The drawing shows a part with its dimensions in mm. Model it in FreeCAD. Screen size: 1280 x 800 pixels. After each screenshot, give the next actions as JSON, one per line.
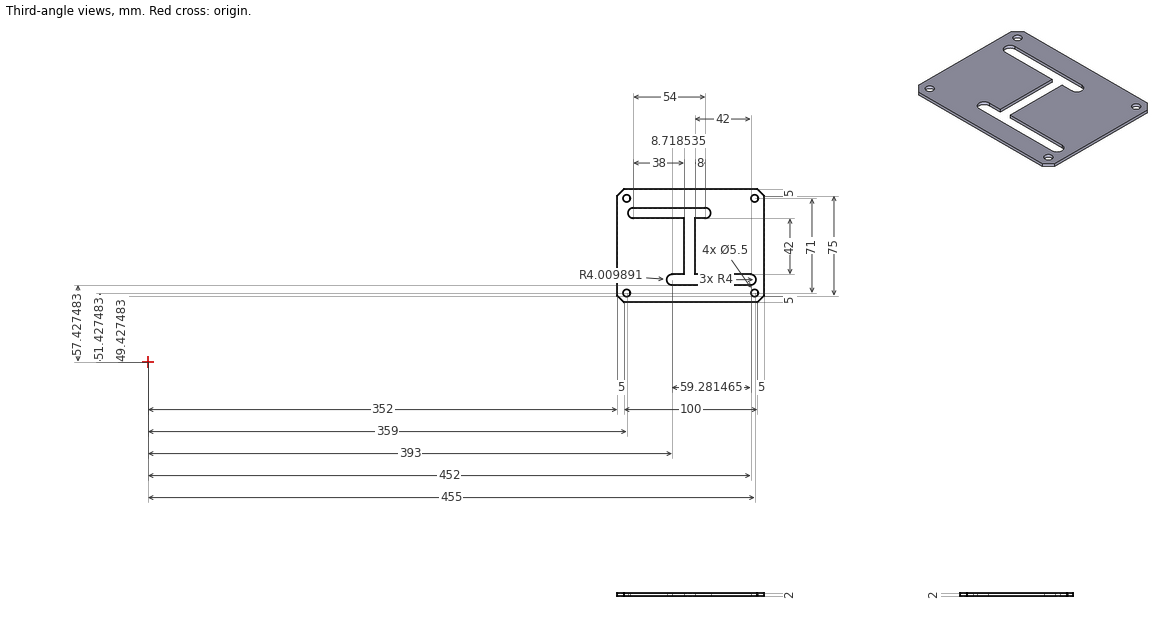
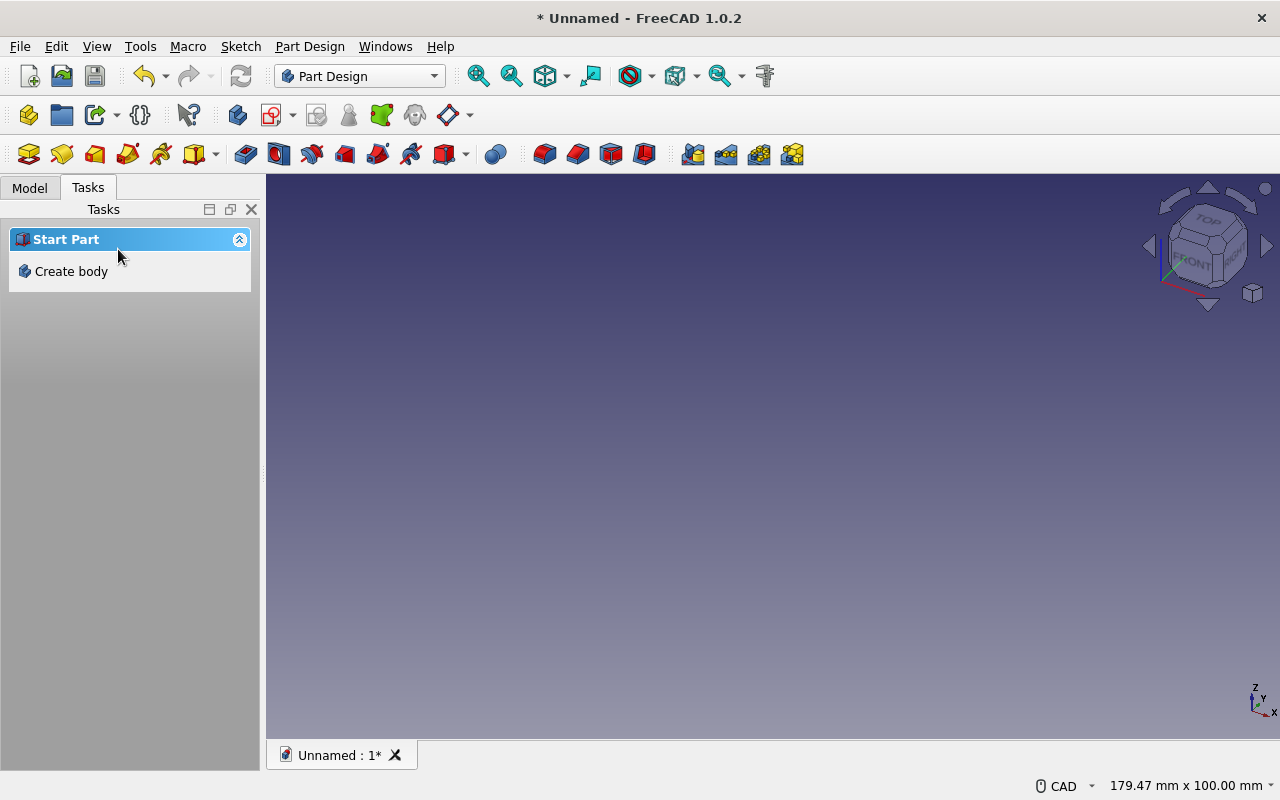
{"action": "key", "text": "v f"}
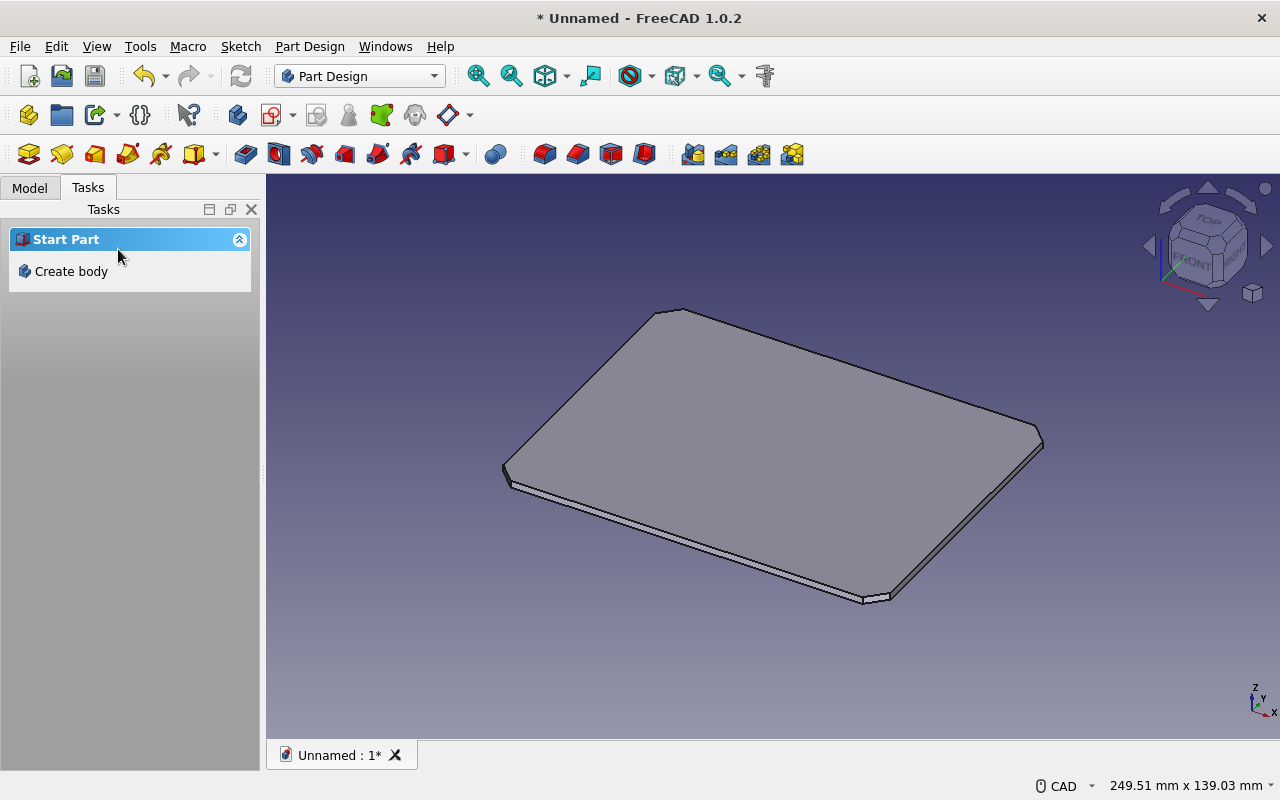
{"action": "left_click", "coordinate": [773, 452]}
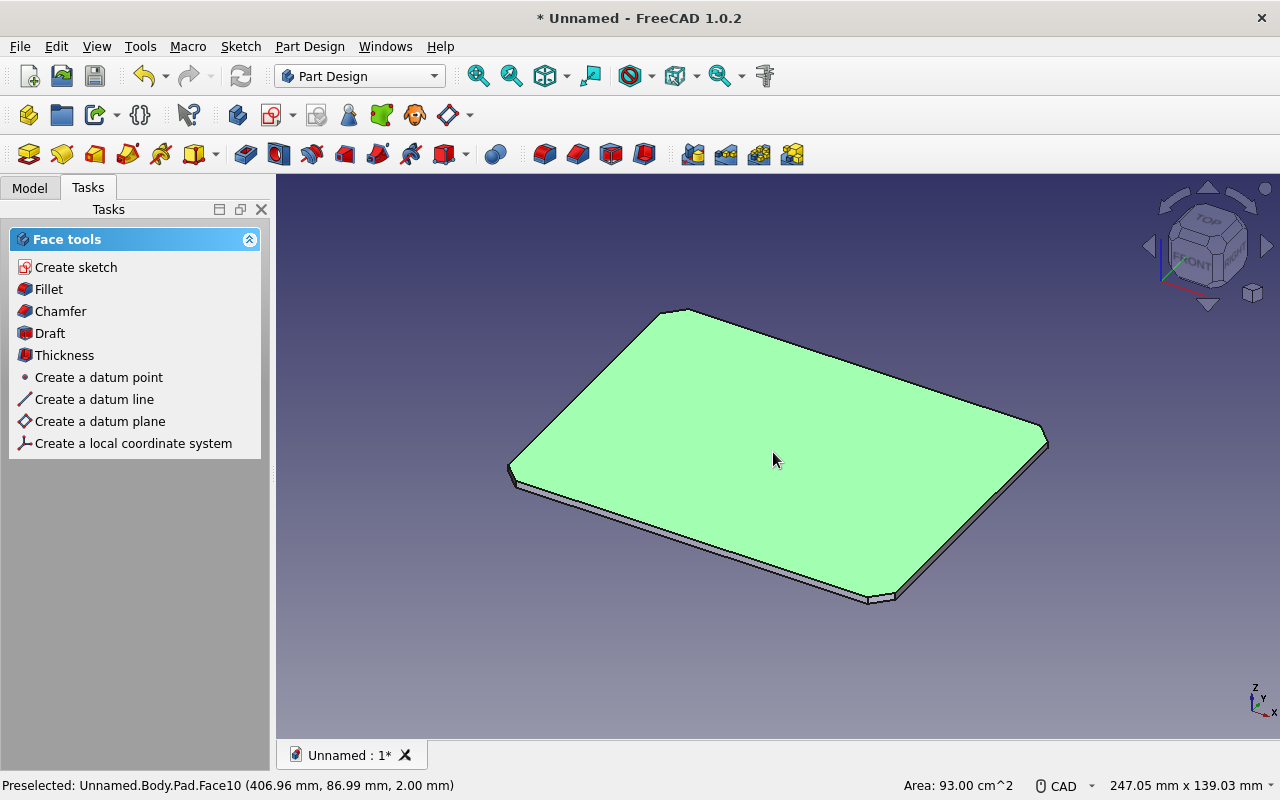
{"action": "left_click", "coordinate": [270, 116]}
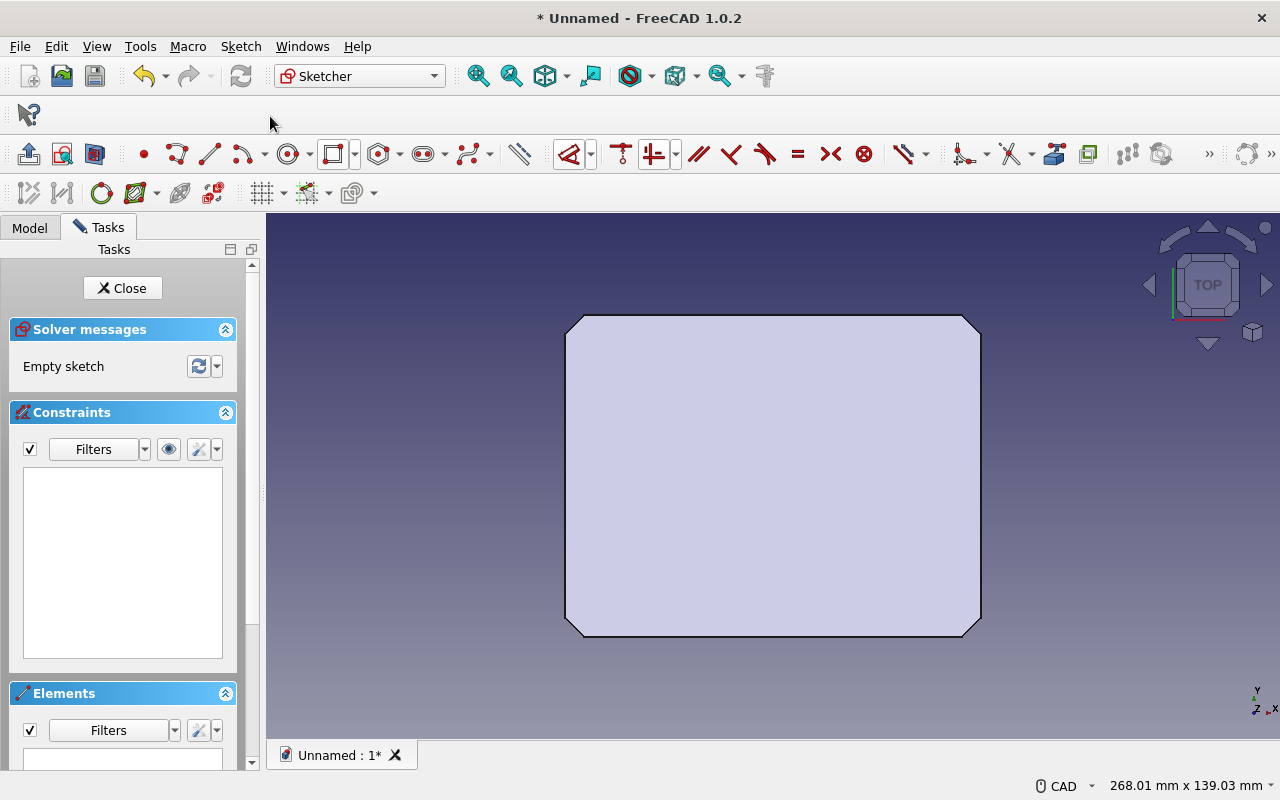
{"action": "scroll", "coordinate": [924, 482], "scroll_direction": "up", "scroll_amount": 2}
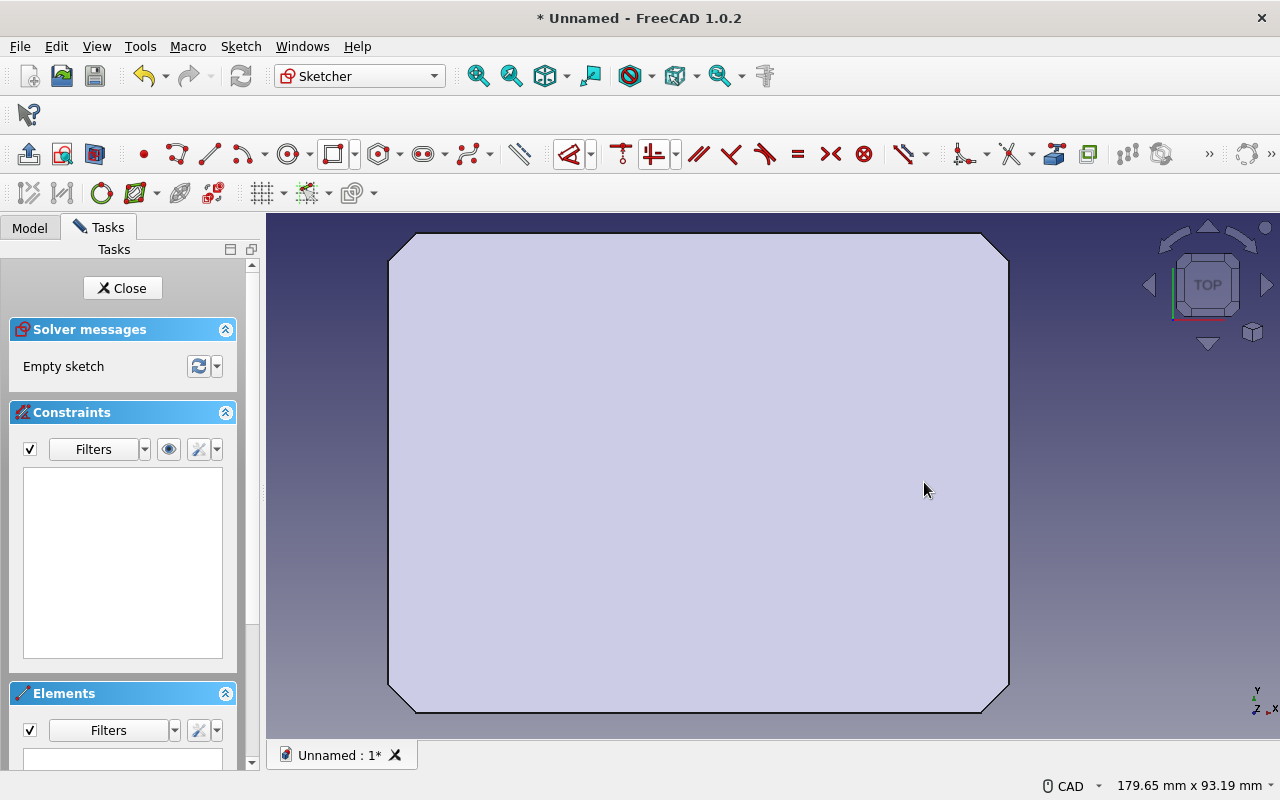
{"action": "left_click", "coordinate": [210, 154]}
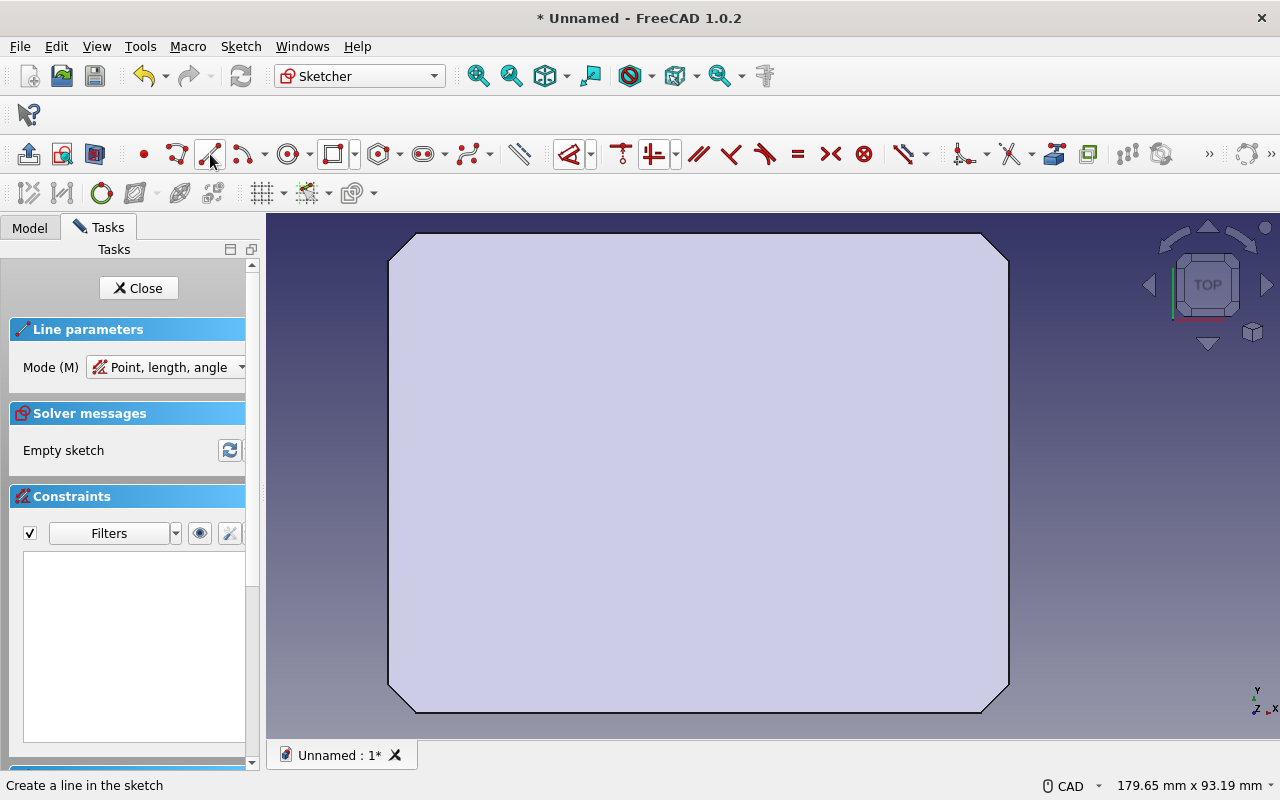
{"action": "left_click", "coordinate": [618, 639]}
{"action": "left_click", "coordinate": [952, 639]}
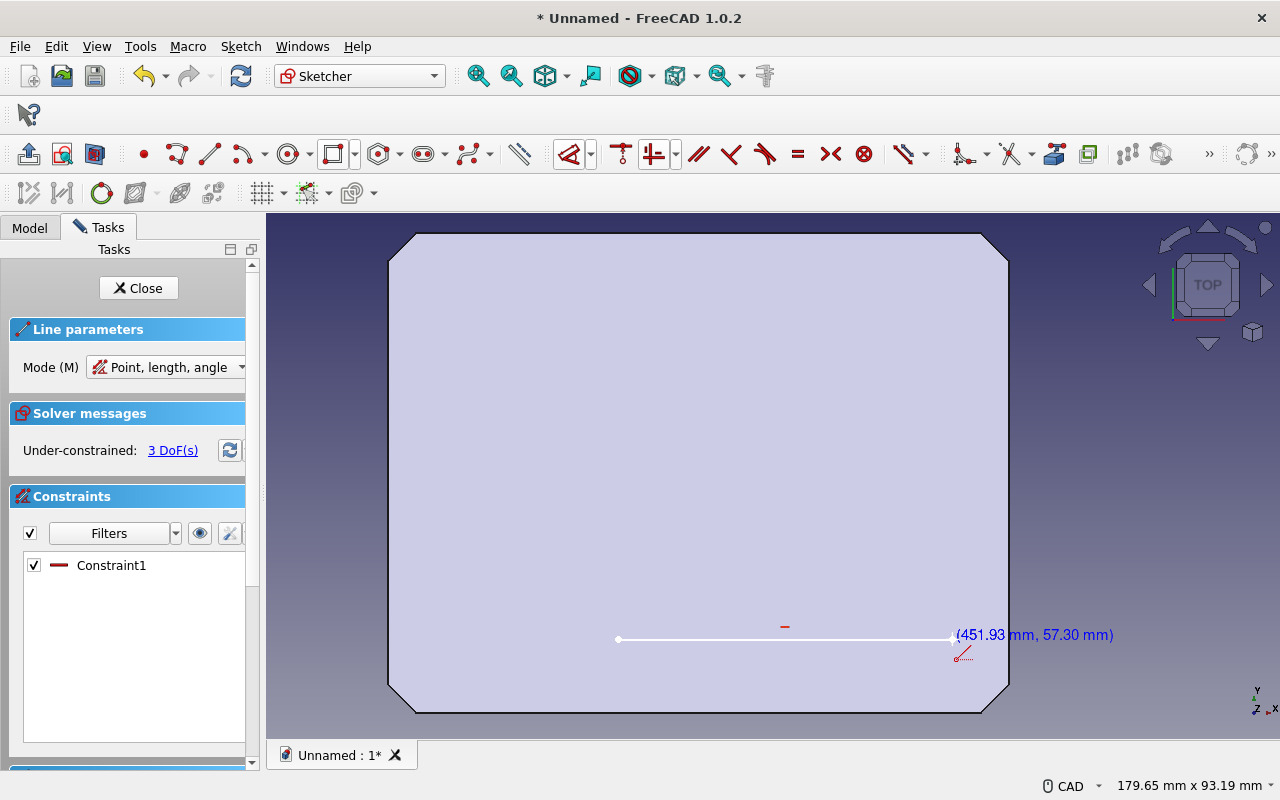
{"action": "left_click", "coordinate": [177, 154]}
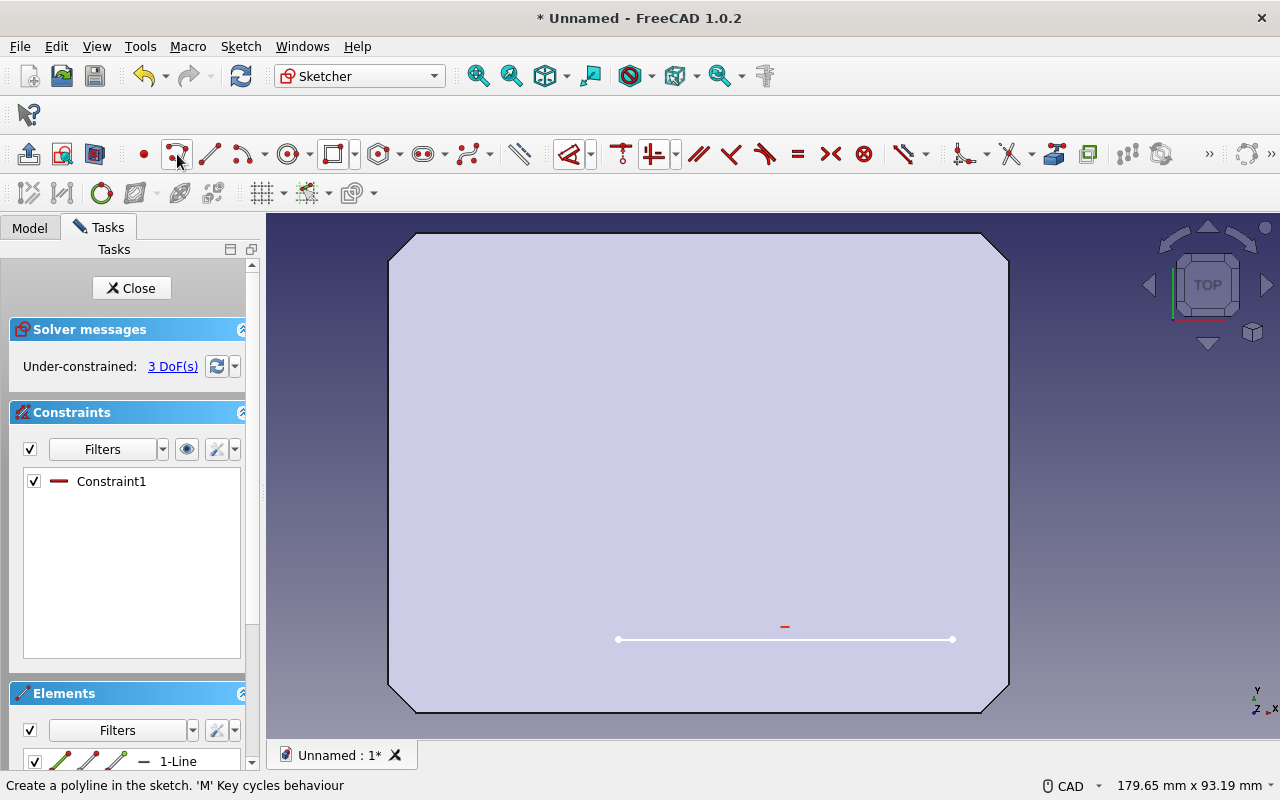
{"action": "left_click", "coordinate": [952, 594]}
{"action": "left_click", "coordinate": [715, 594]}
{"action": "left_click", "coordinate": [715, 357]}
{"action": "left_click", "coordinate": [761, 357]}
{"action": "right_click", "coordinate": [761, 357]}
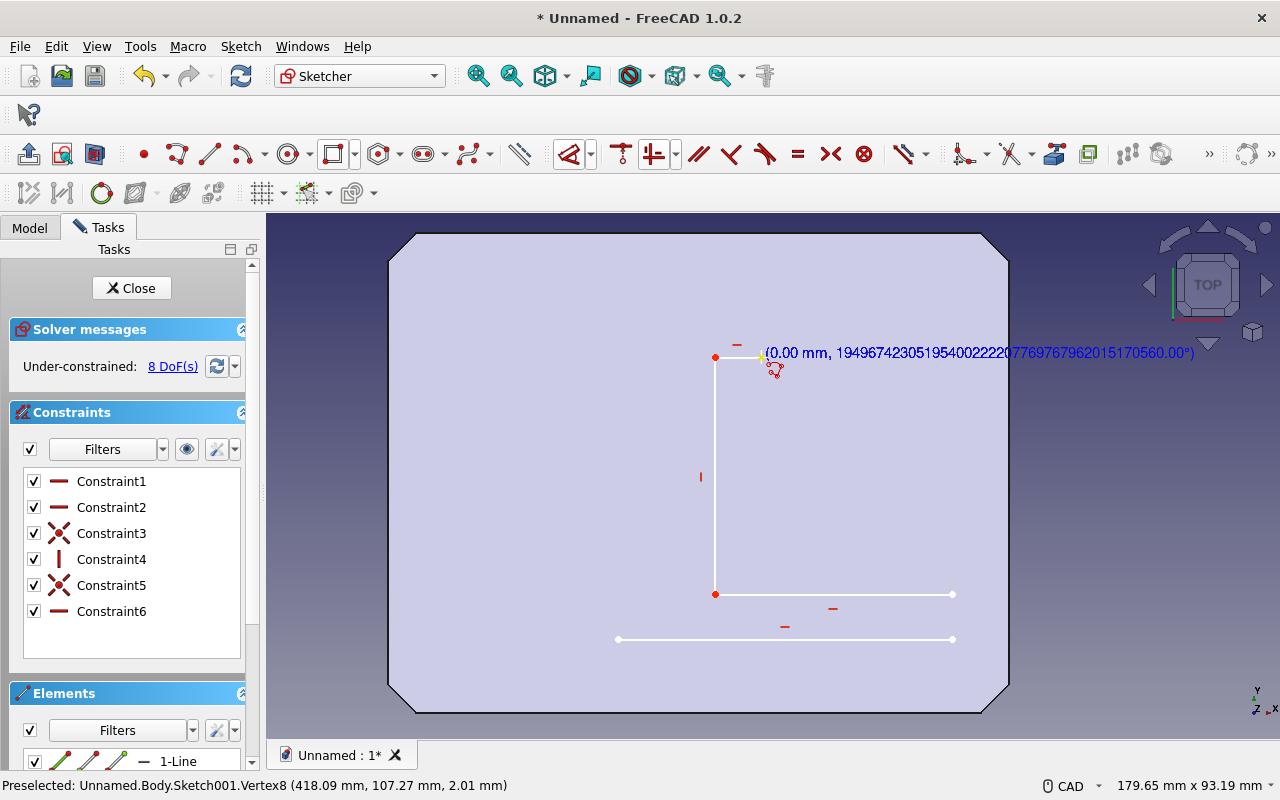
{"action": "left_click", "coordinate": [210, 154]}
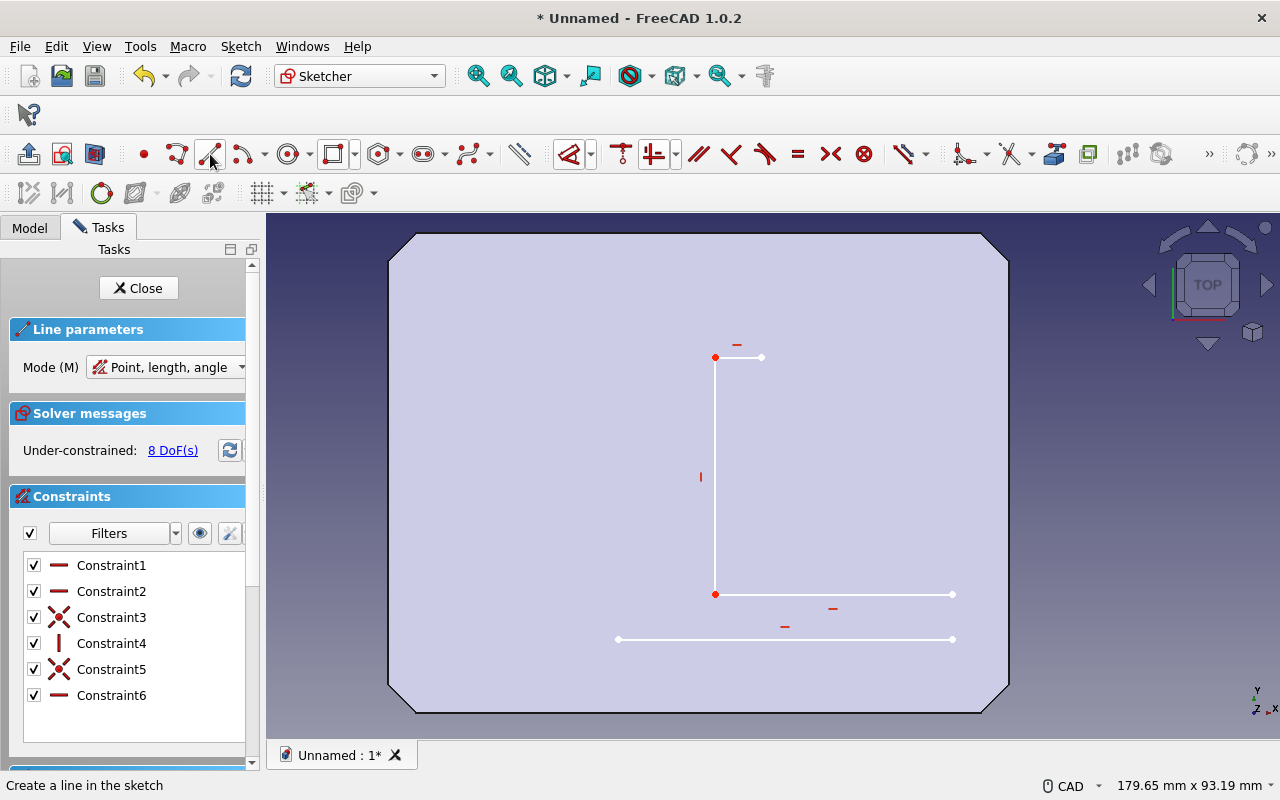
{"action": "left_click", "coordinate": [761, 312]}
{"action": "left_click", "coordinate": [456, 312]}